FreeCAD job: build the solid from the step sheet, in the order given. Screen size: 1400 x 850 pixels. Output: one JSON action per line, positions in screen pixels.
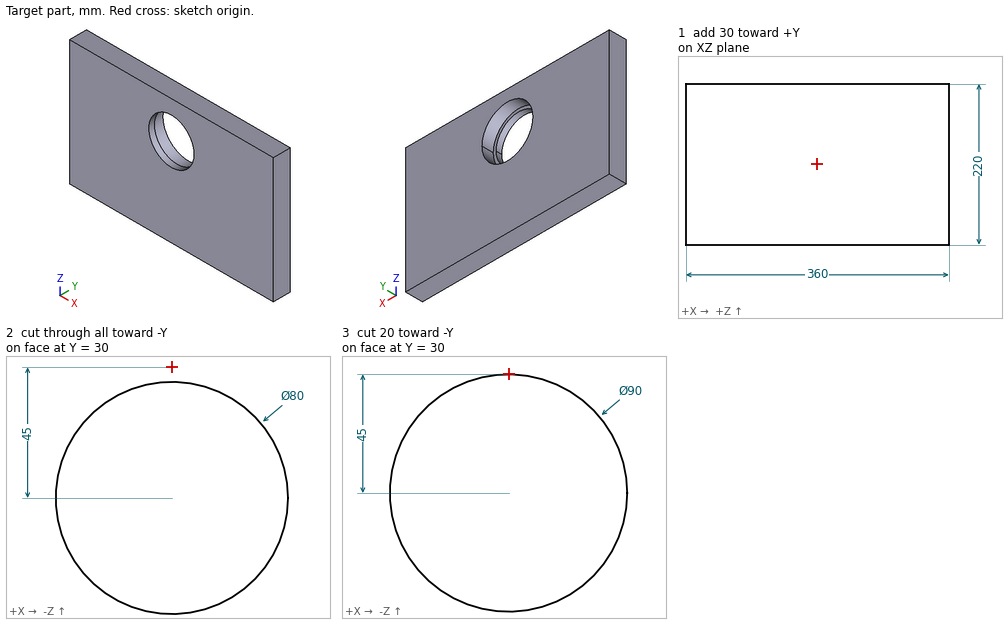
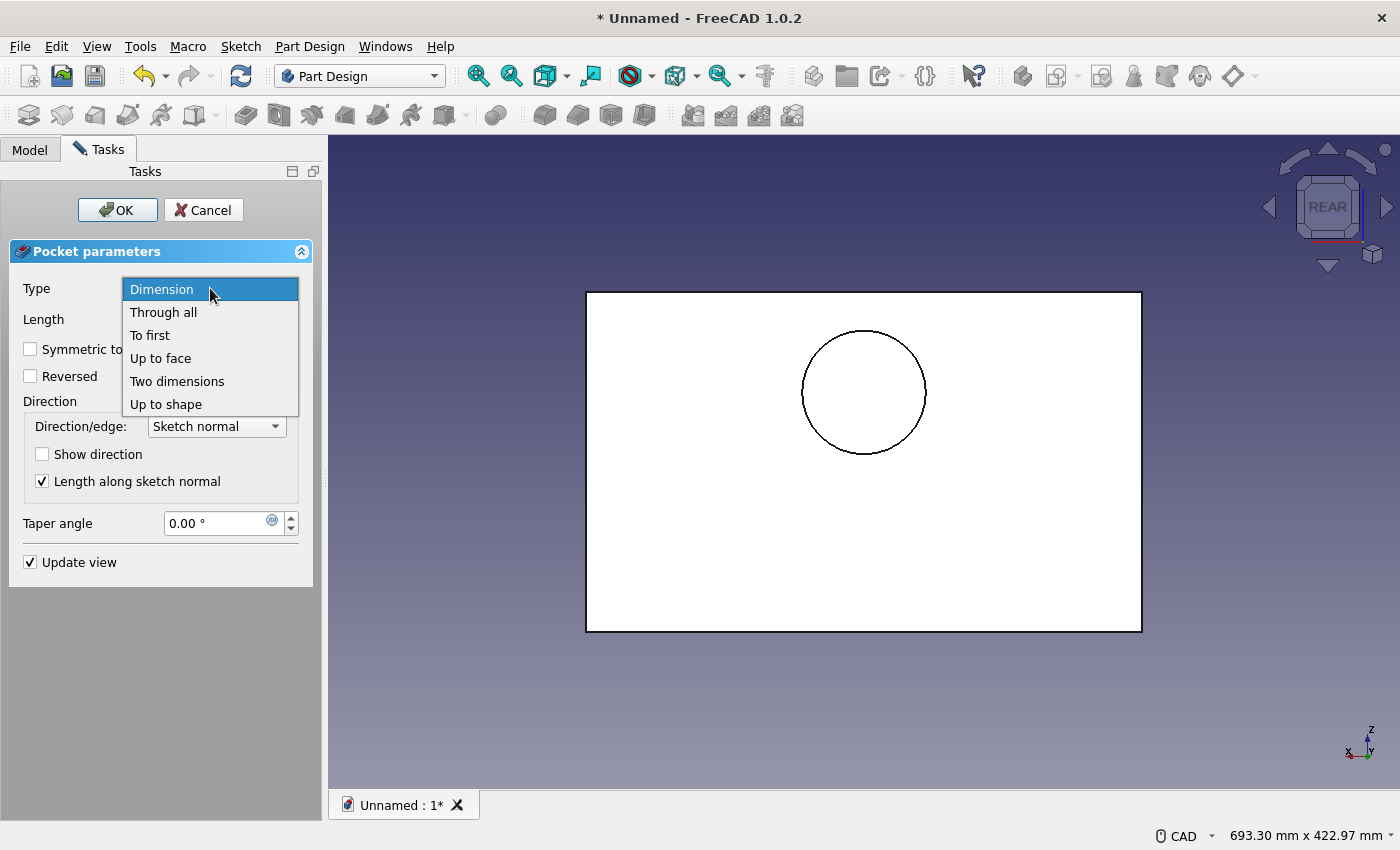
{"action": "left_click", "coordinate": [208, 312]}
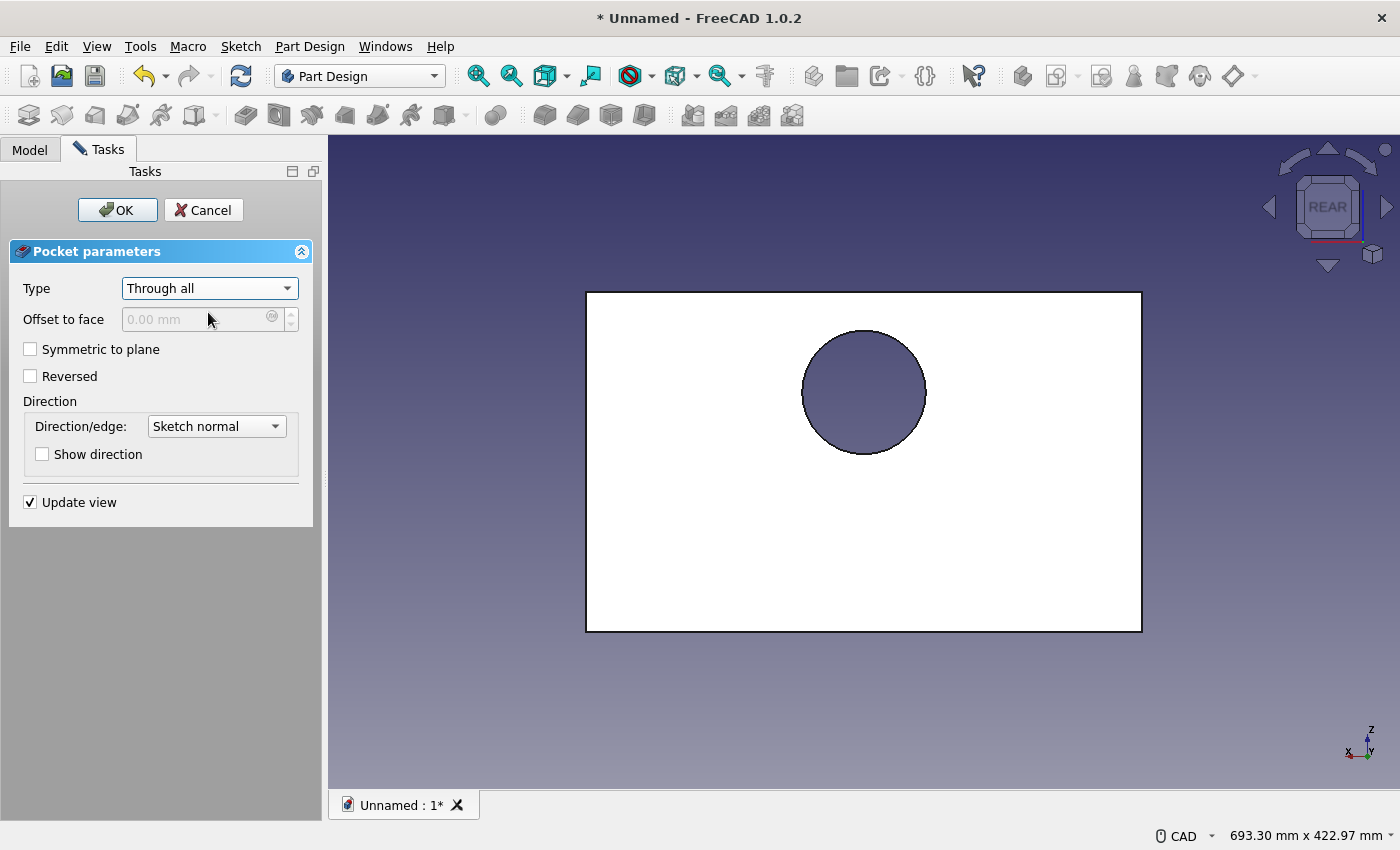
{"action": "left_click", "coordinate": [118, 210]}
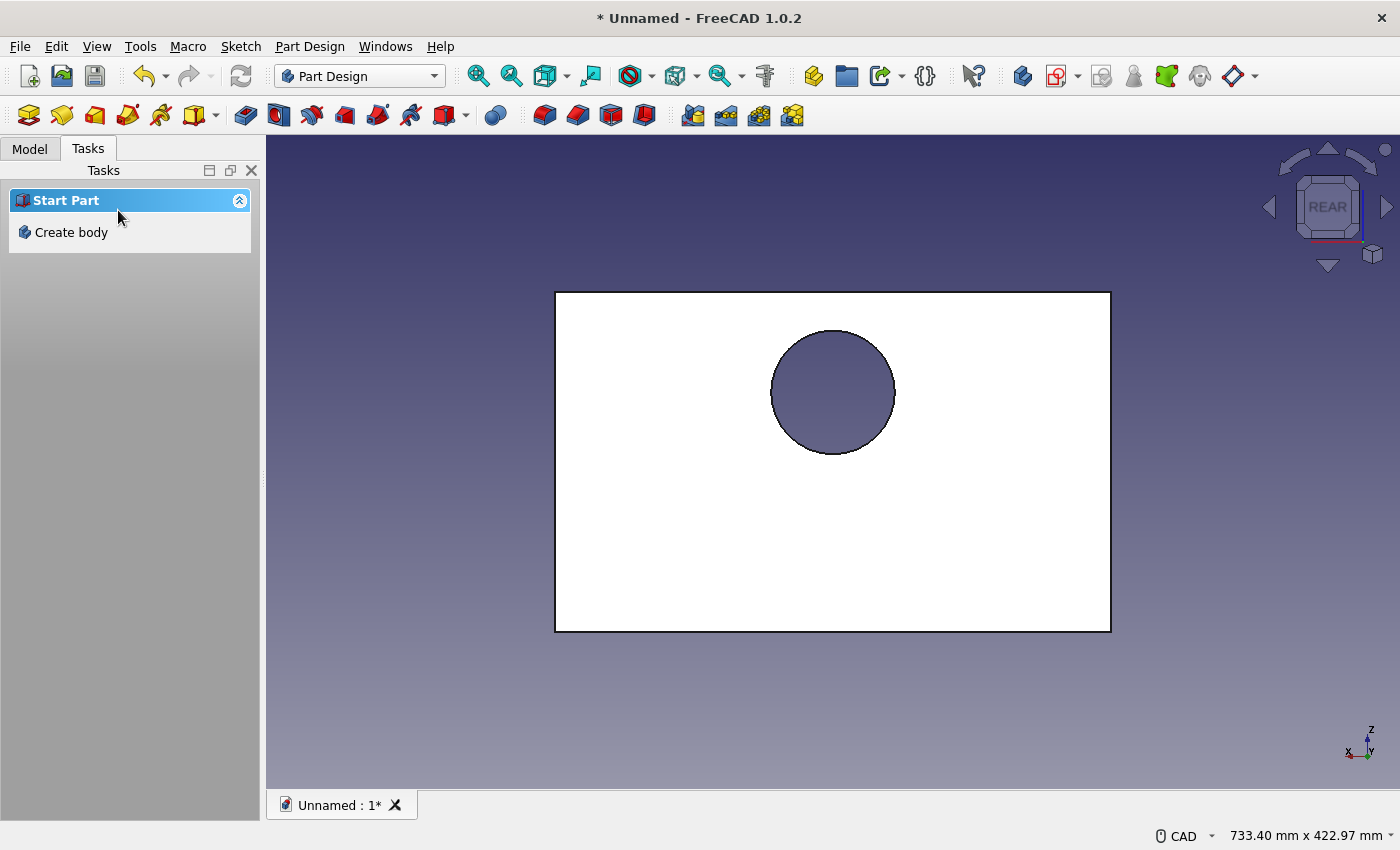
{"action": "left_click", "coordinate": [674, 510]}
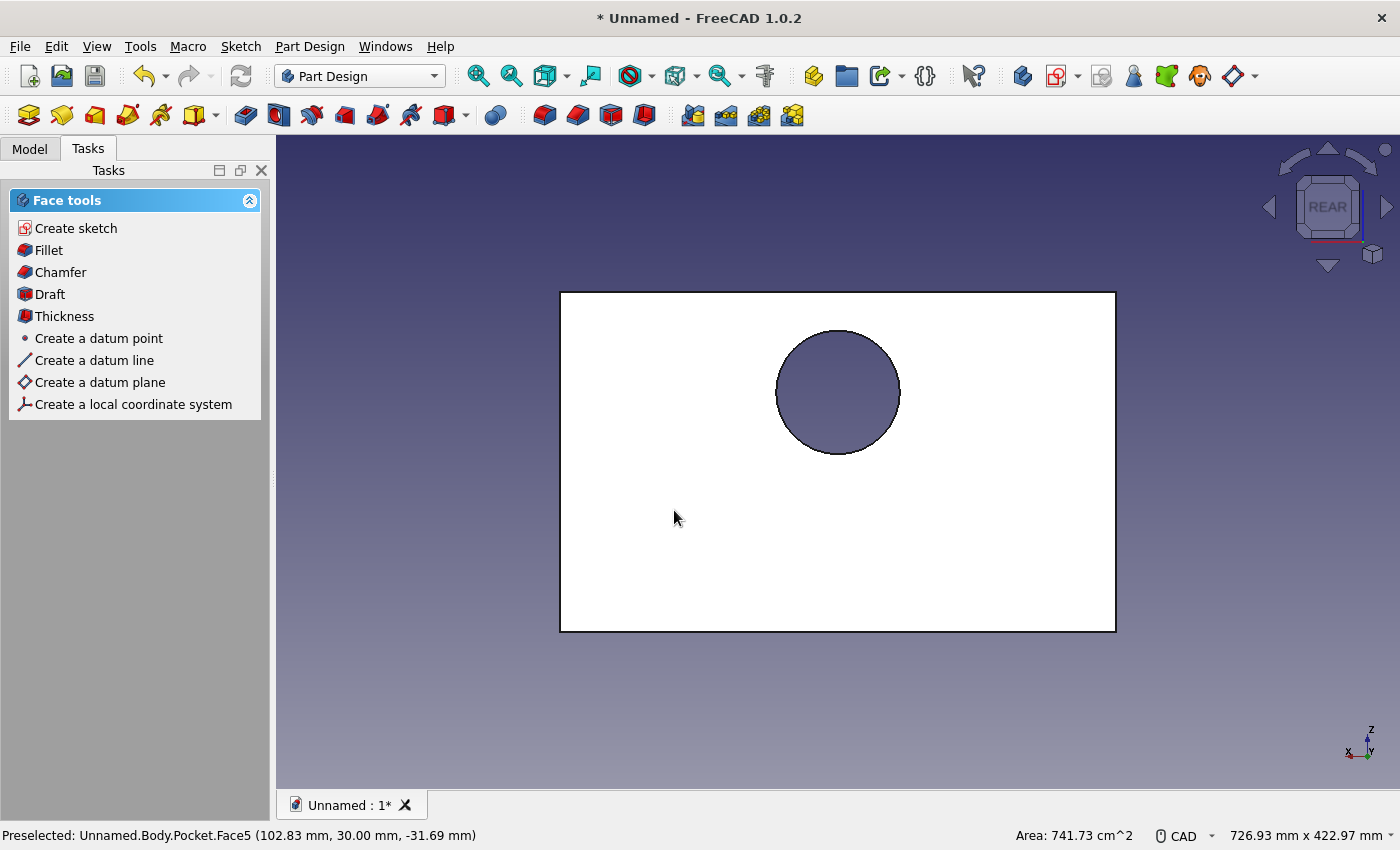
{"action": "left_click", "coordinate": [1056, 76]}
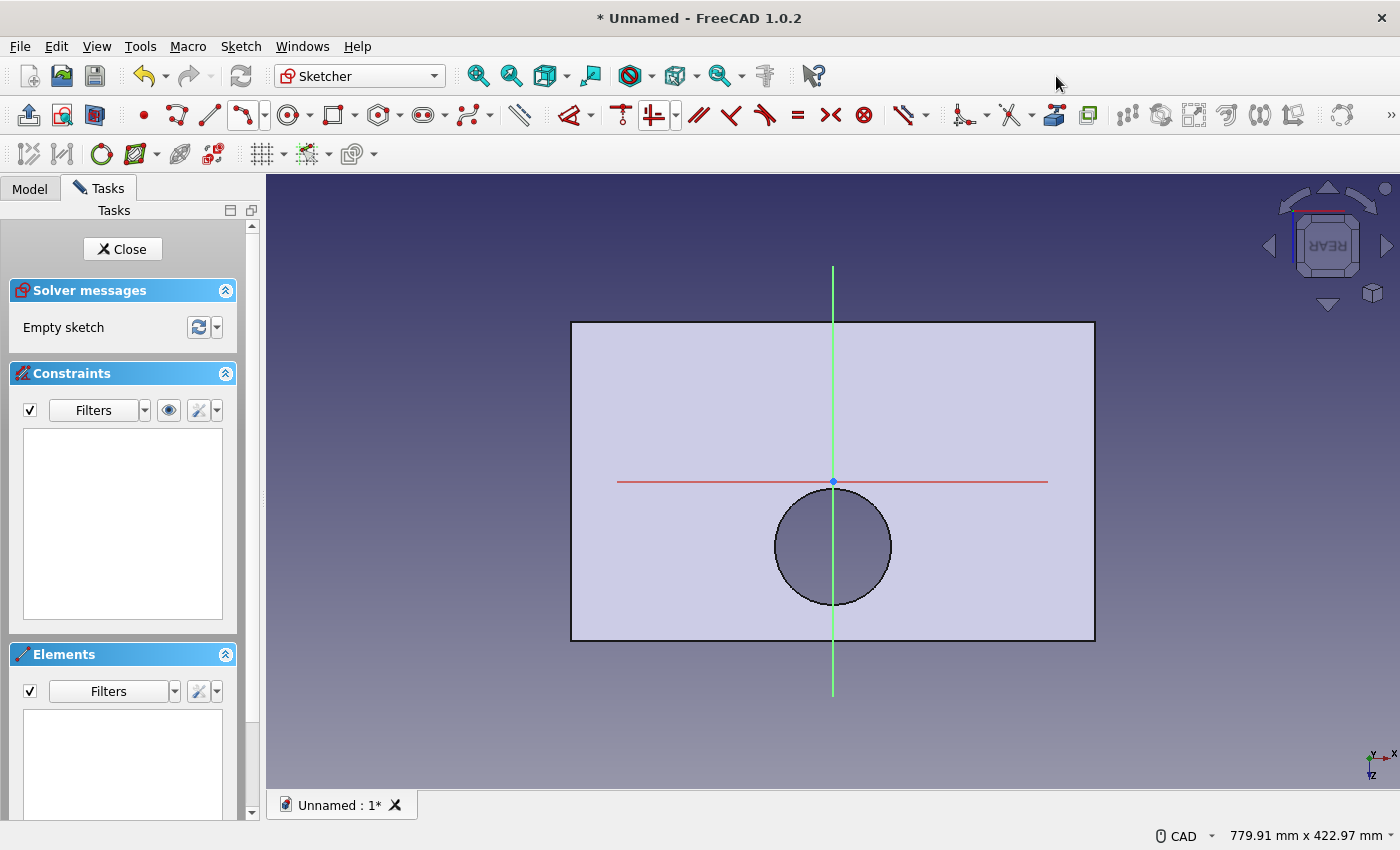
{"action": "scroll", "coordinate": [863, 575], "scroll_direction": "up", "scroll_amount": 6}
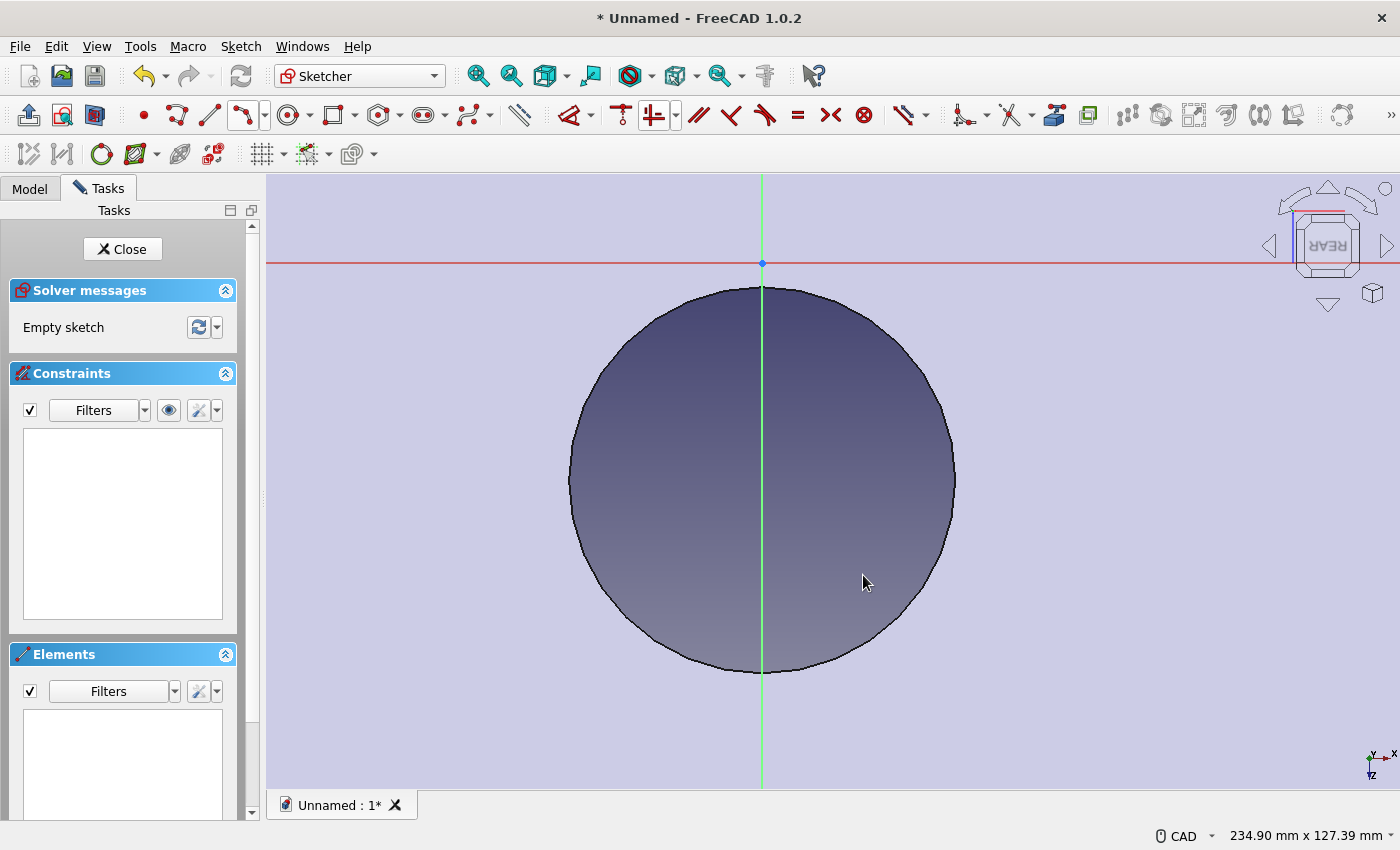
{"action": "left_click", "coordinate": [288, 116]}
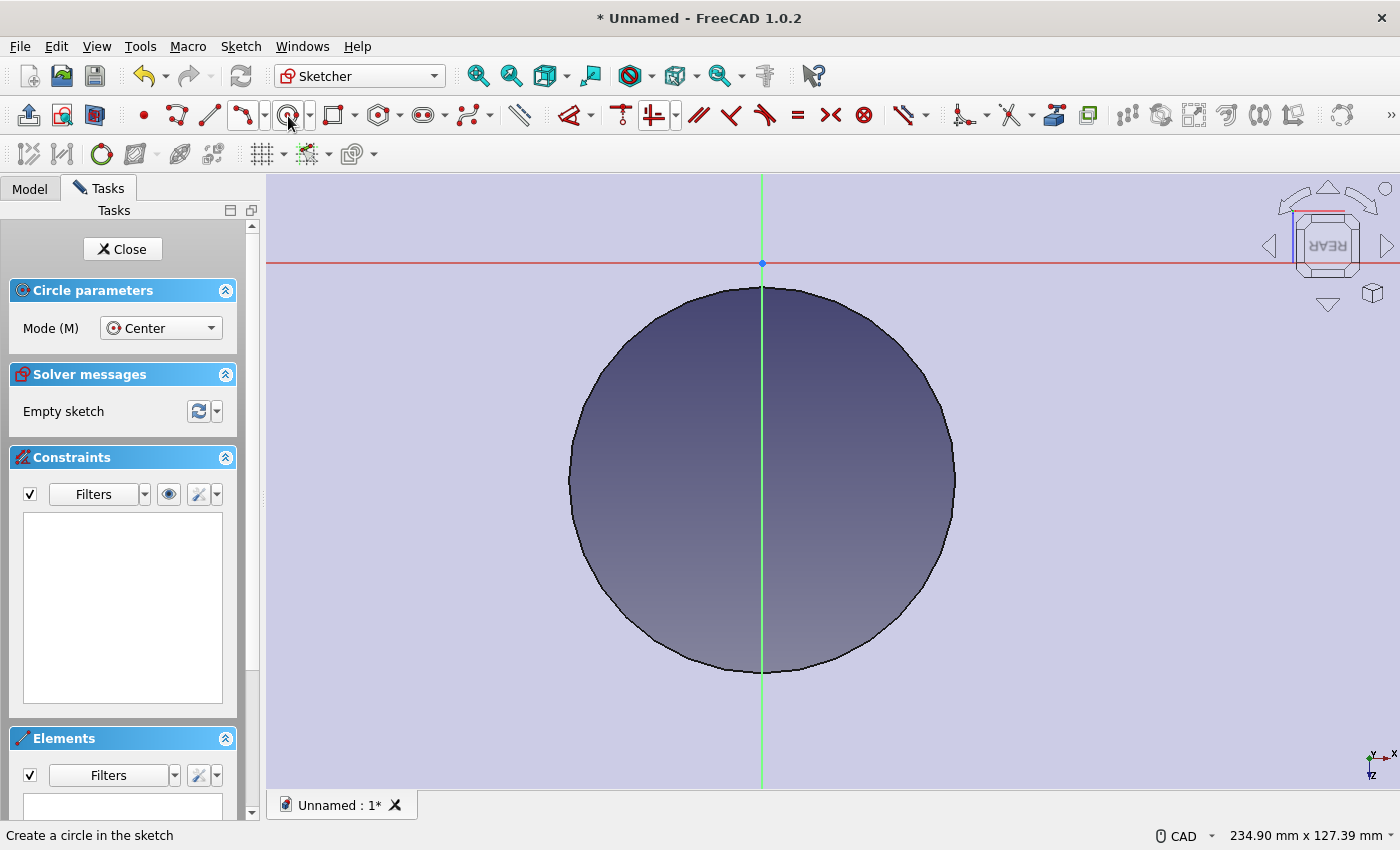
{"action": "left_click", "coordinate": [762, 480]}
{"action": "mouse_move", "coordinate": [916, 327]}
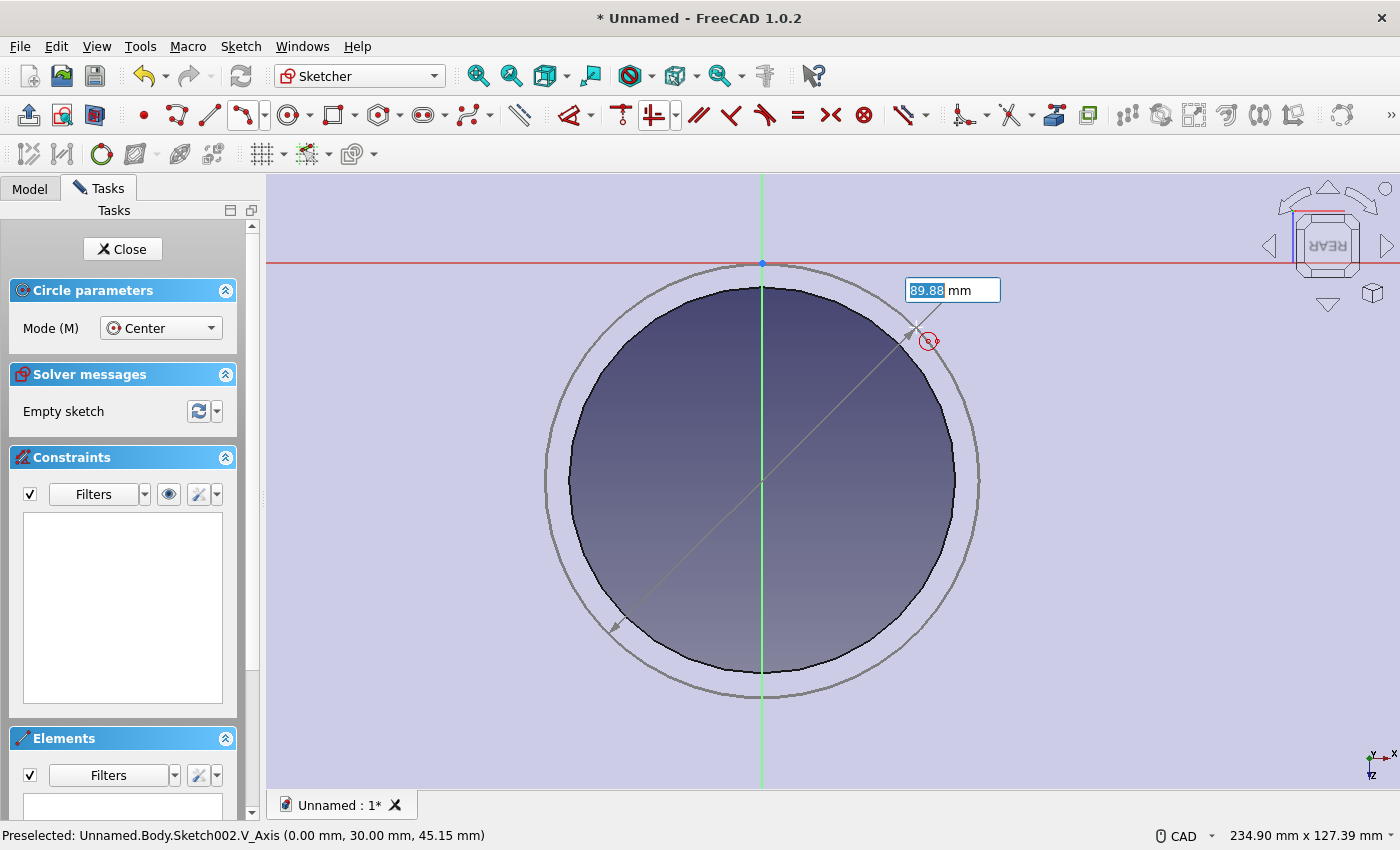
{"action": "type", "text": "90"}
{"action": "key", "text": "Return"}
{"action": "key", "text": "Escape"}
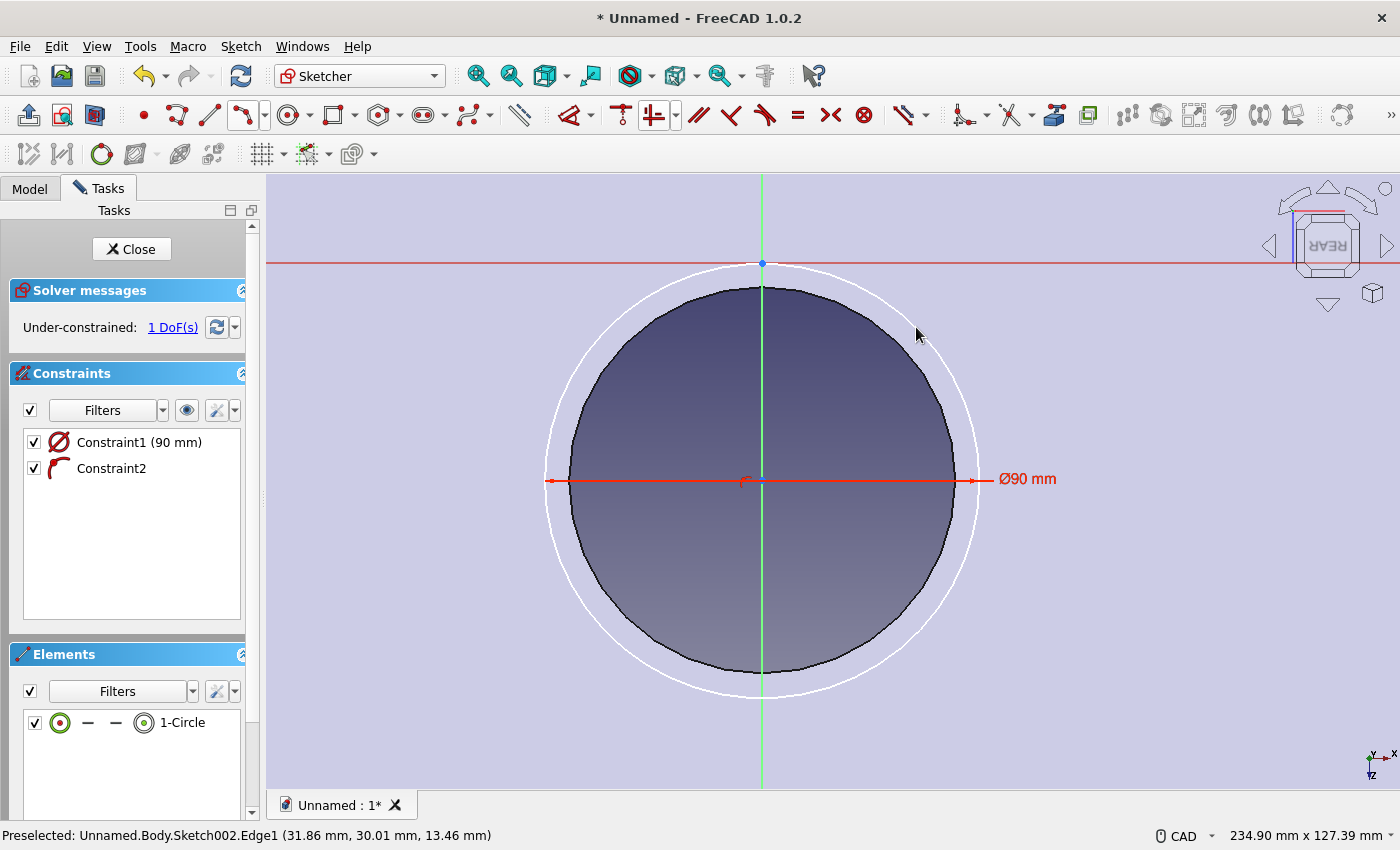
{"action": "left_click", "coordinate": [568, 116]}